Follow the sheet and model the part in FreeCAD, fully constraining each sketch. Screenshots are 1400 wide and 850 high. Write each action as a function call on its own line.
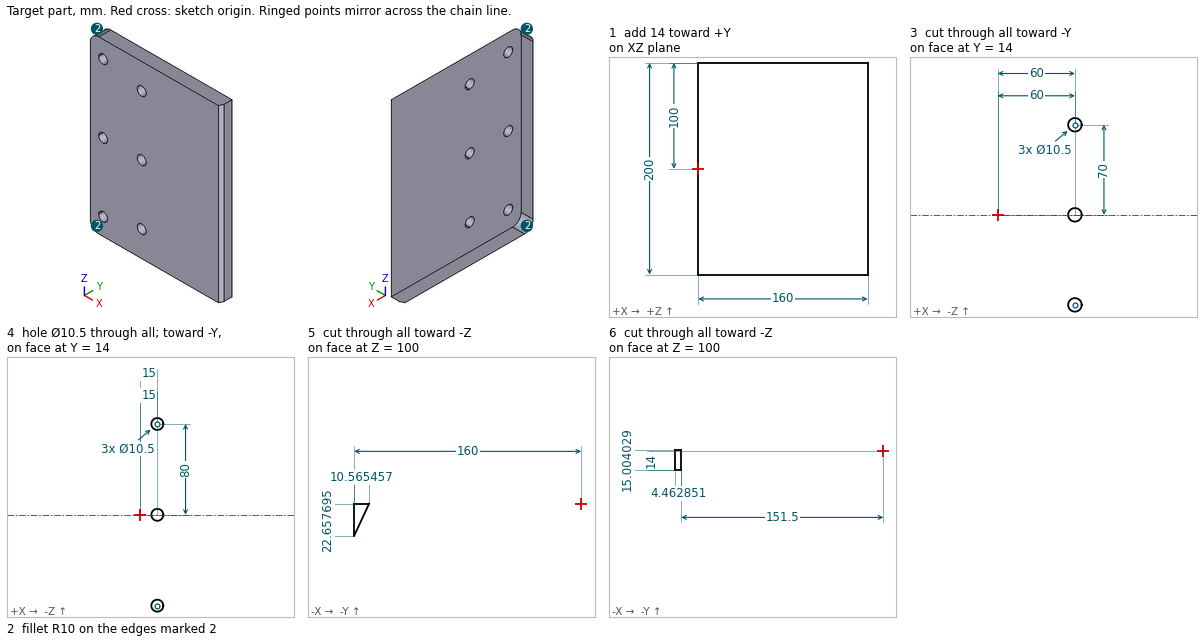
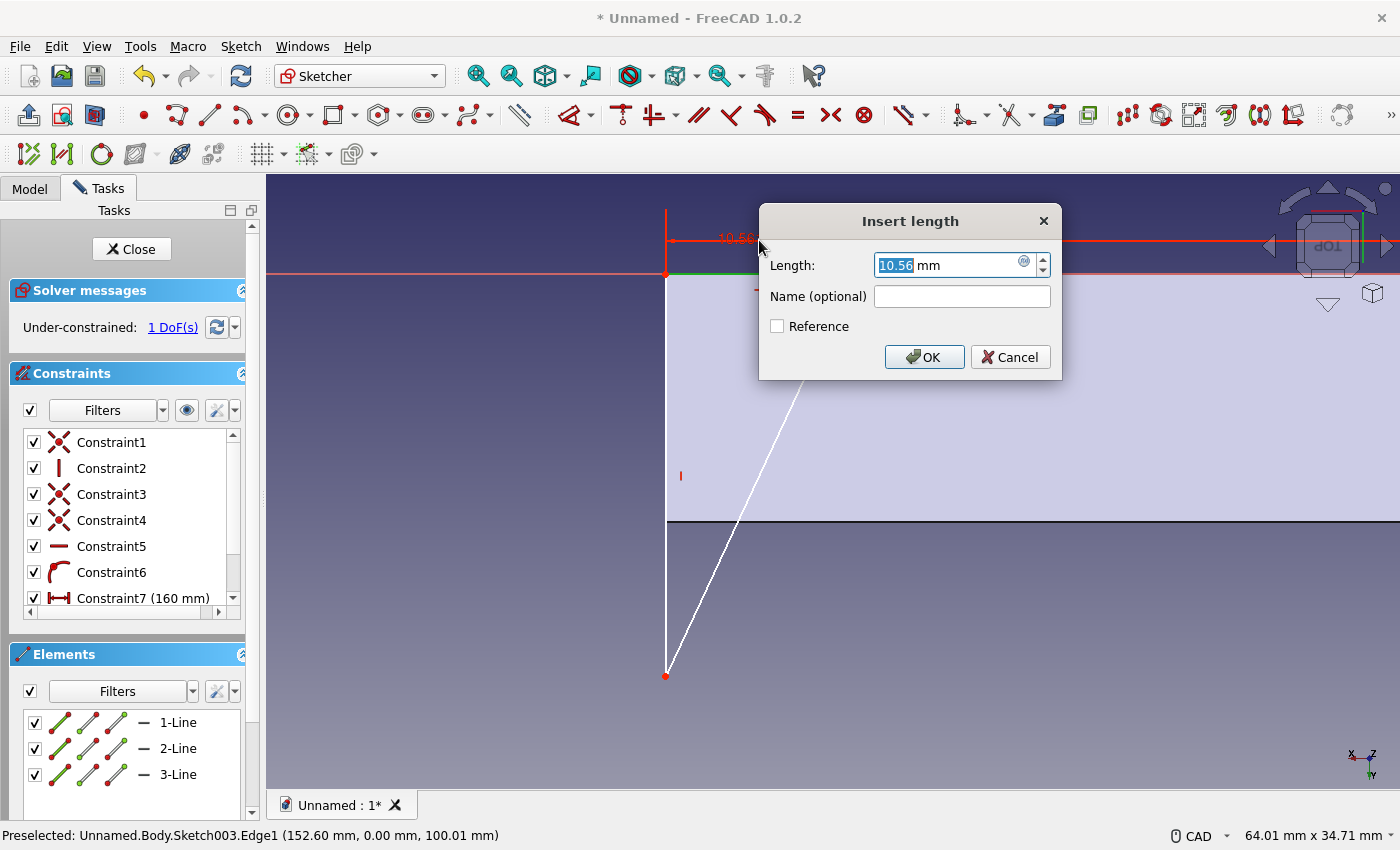
text(10.565457)
key(Return)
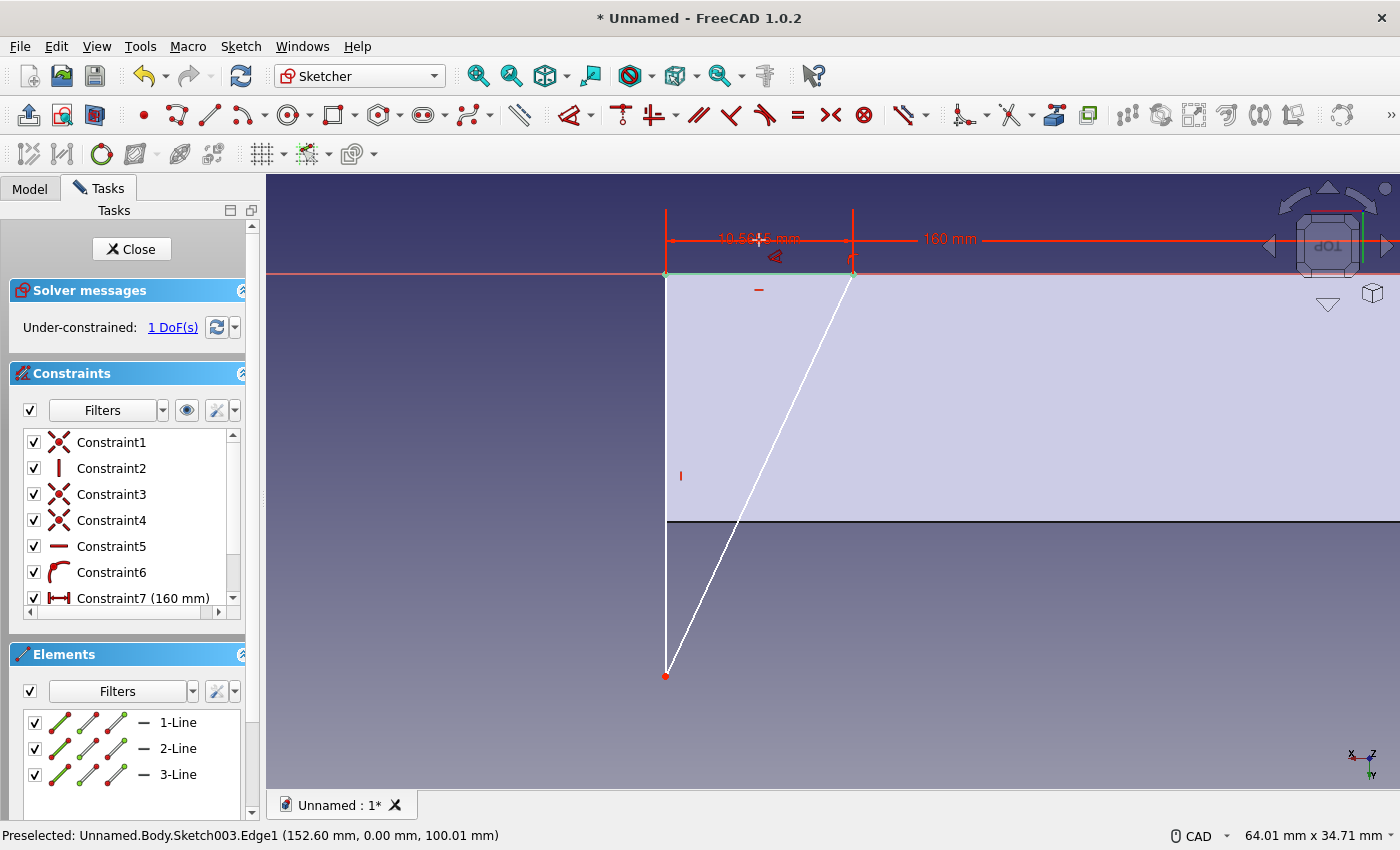
click(666, 395)
click(632, 476)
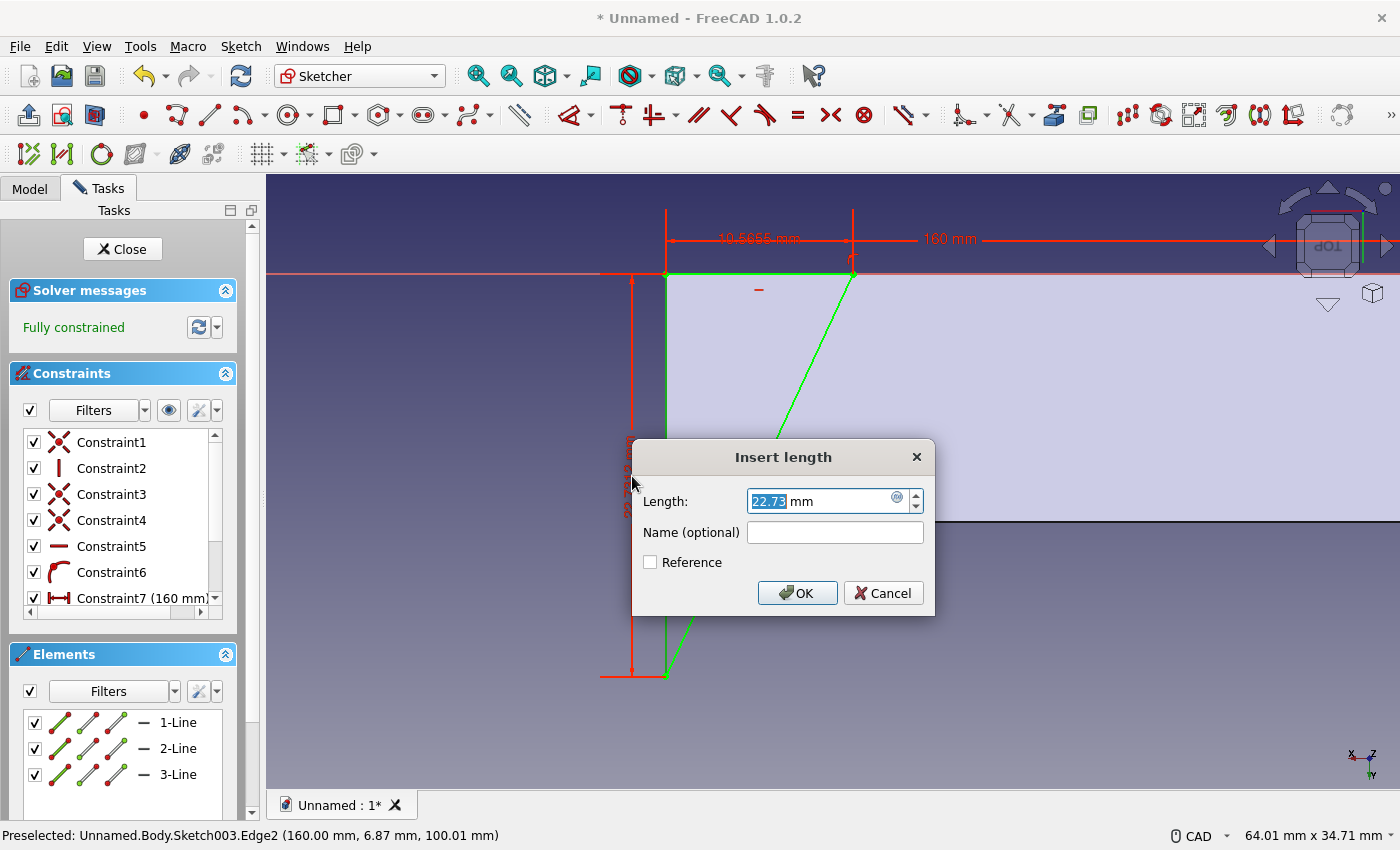
text(22.657695)
key(Return)
key(Escape)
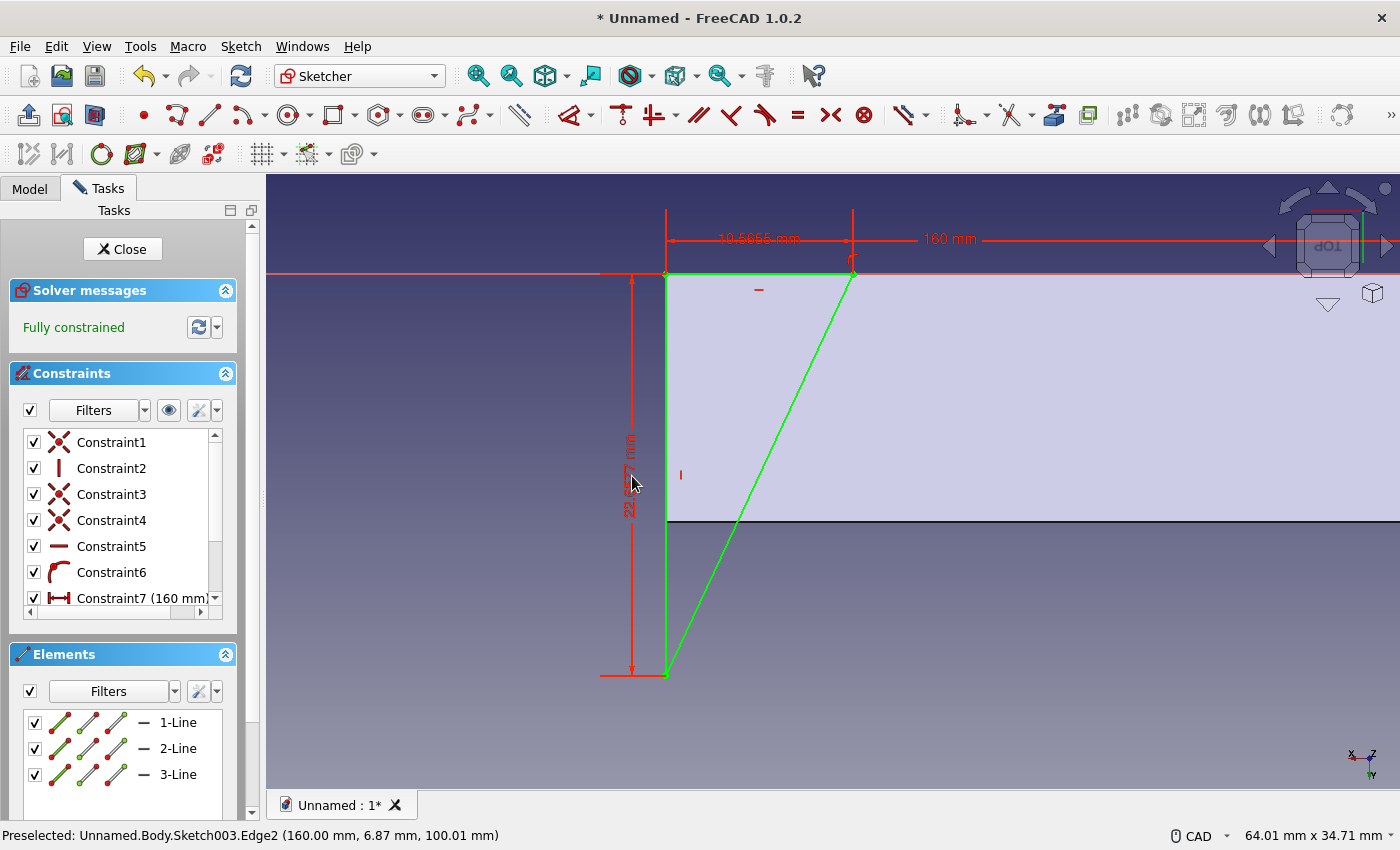
click(123, 249)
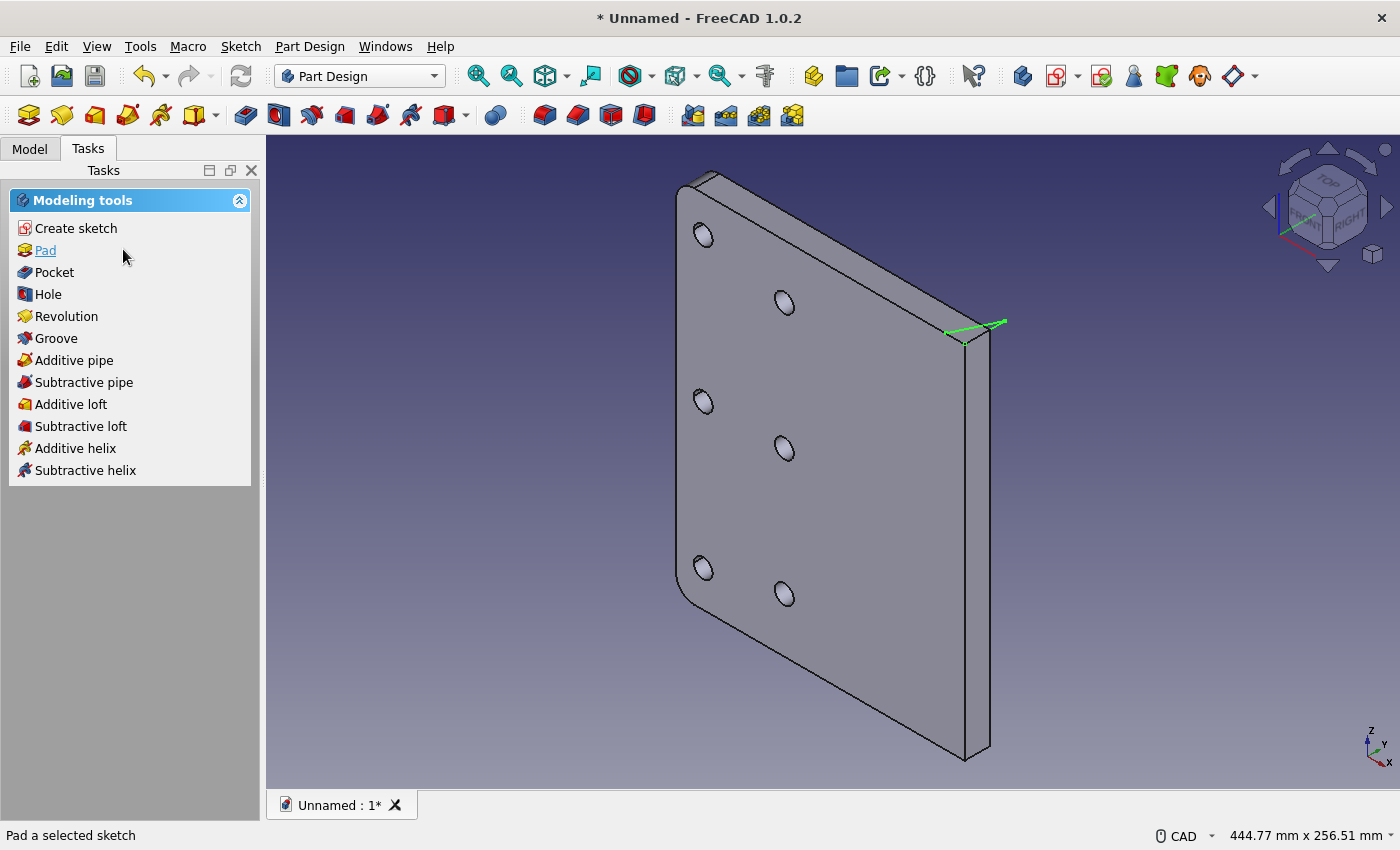
click(246, 116)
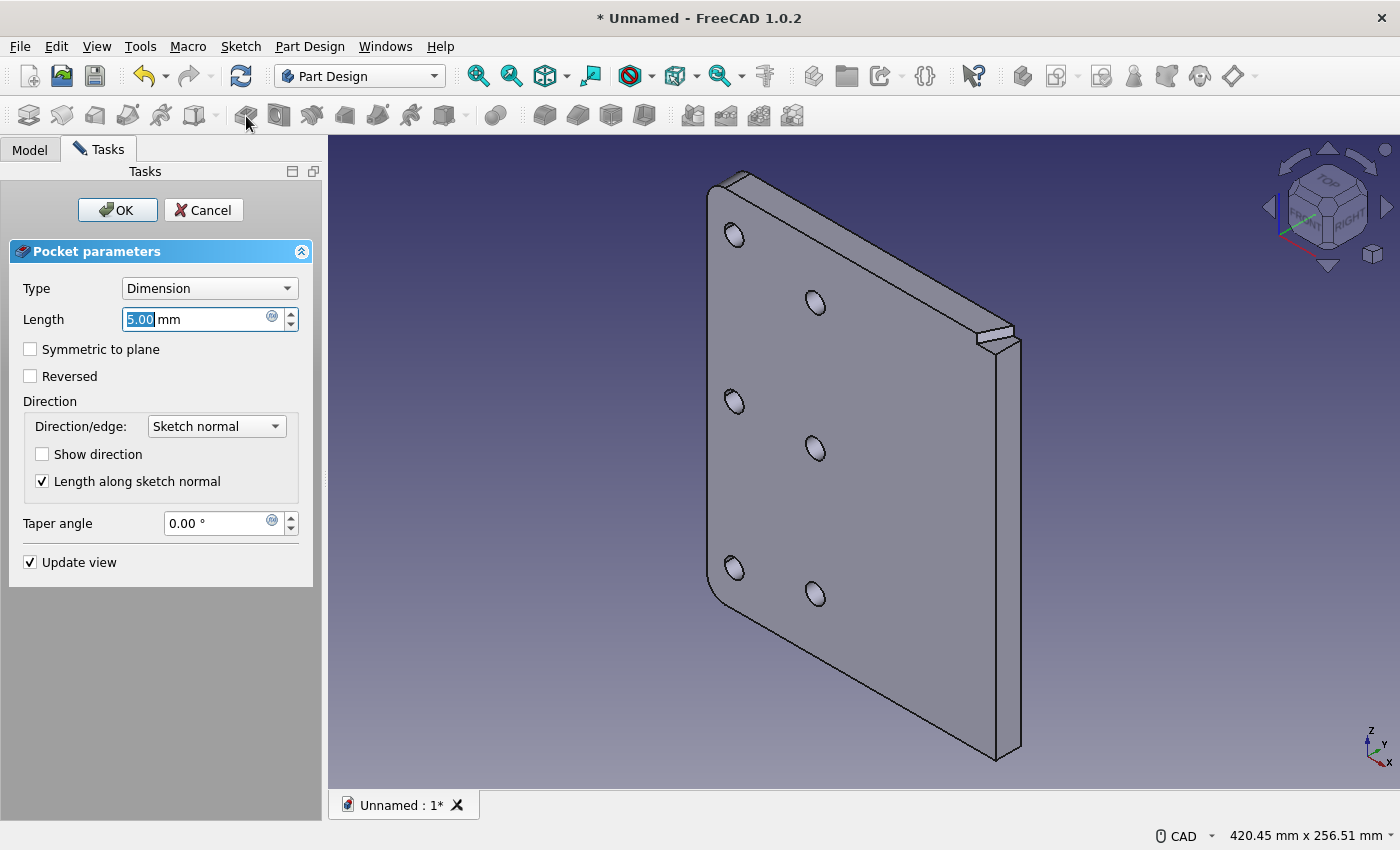
click(210, 288)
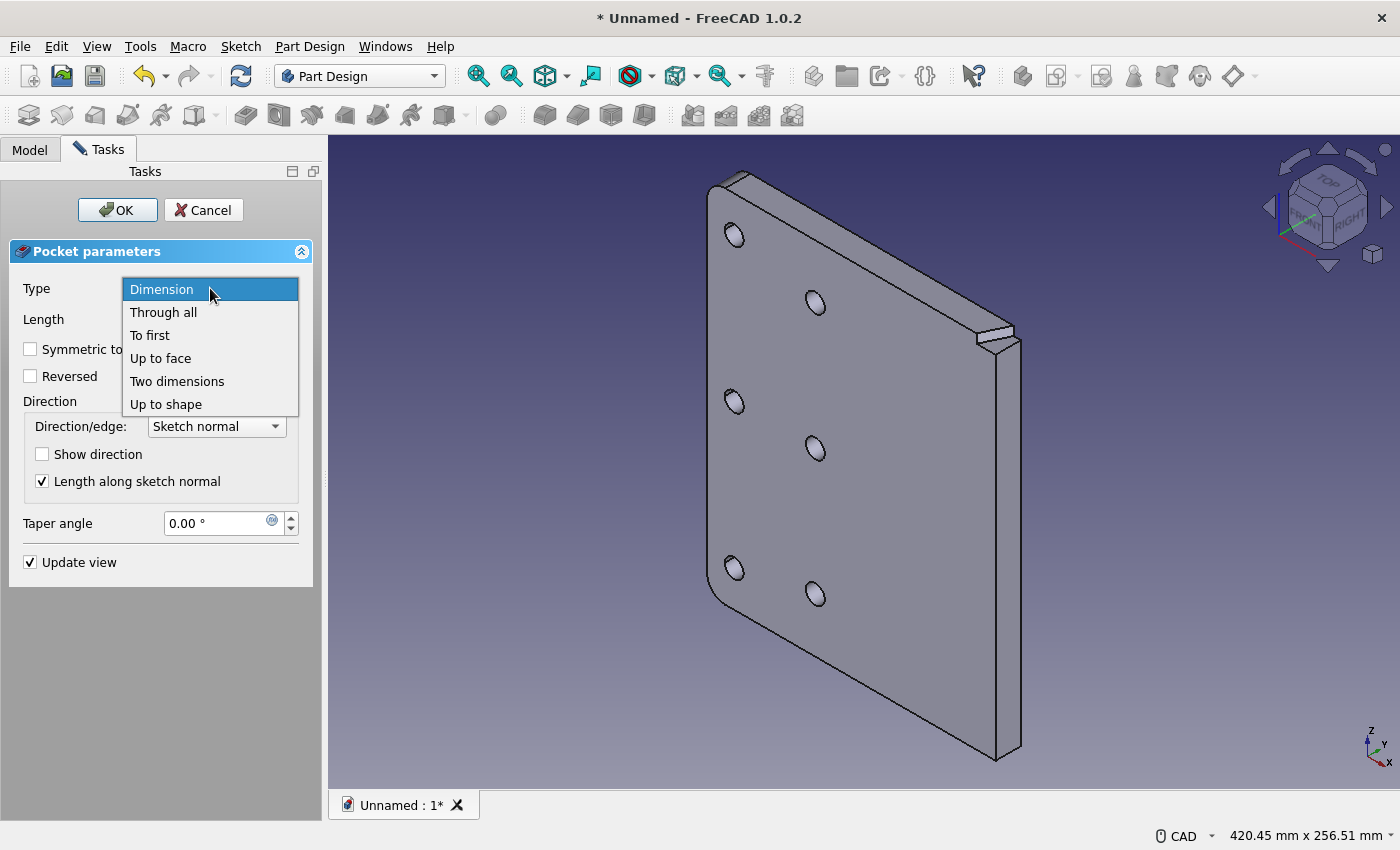
click(208, 312)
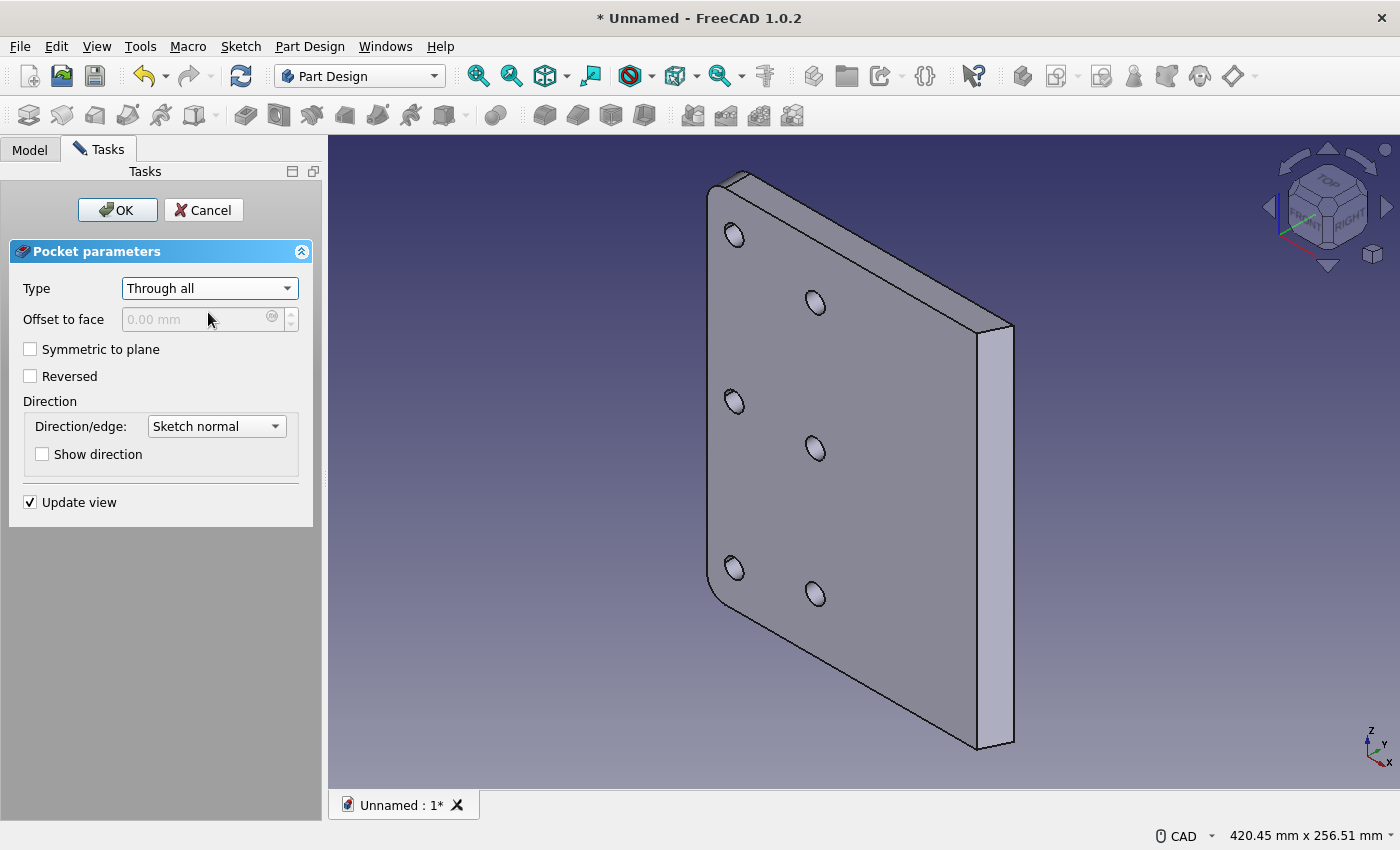
click(118, 210)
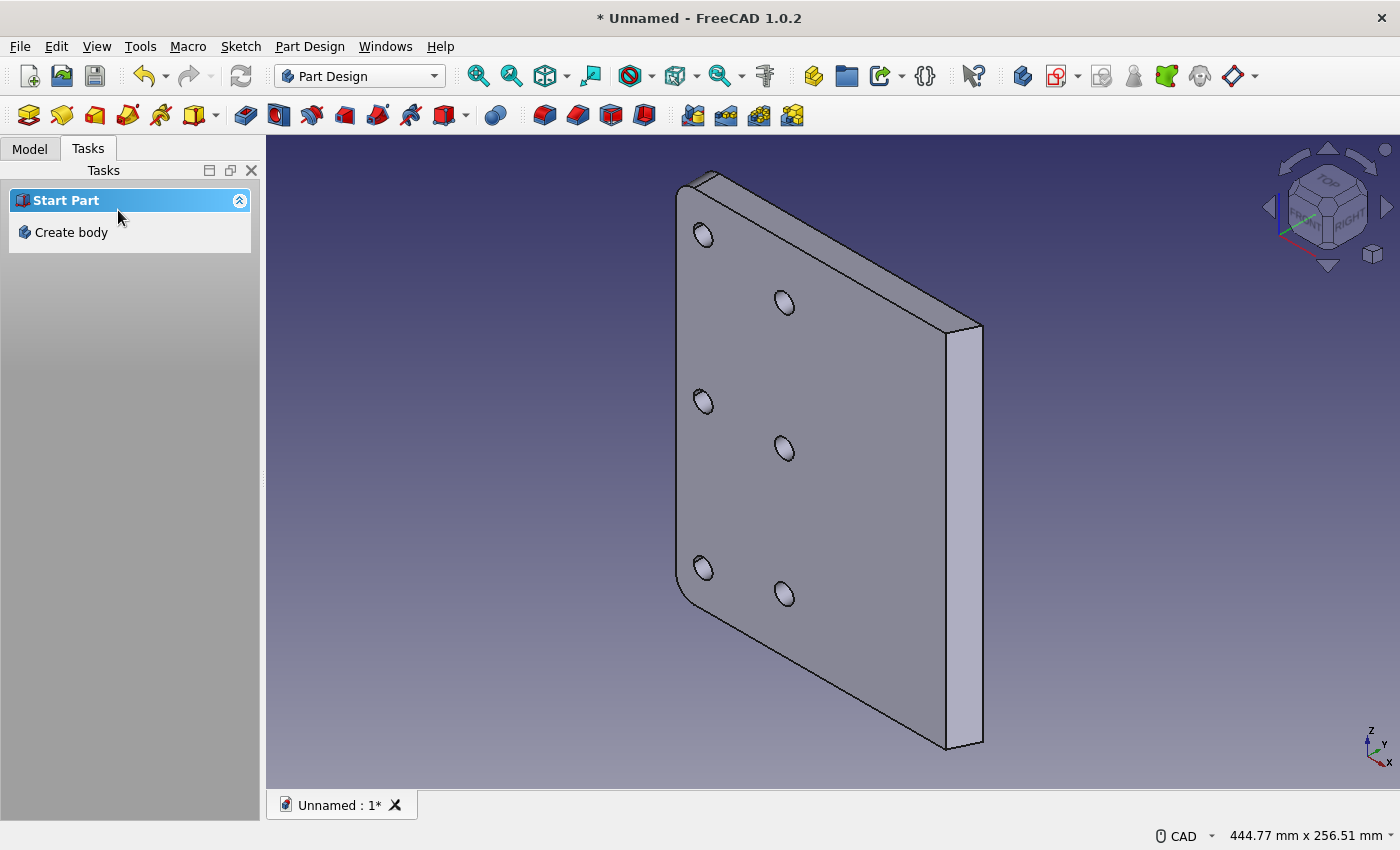
click(914, 299)